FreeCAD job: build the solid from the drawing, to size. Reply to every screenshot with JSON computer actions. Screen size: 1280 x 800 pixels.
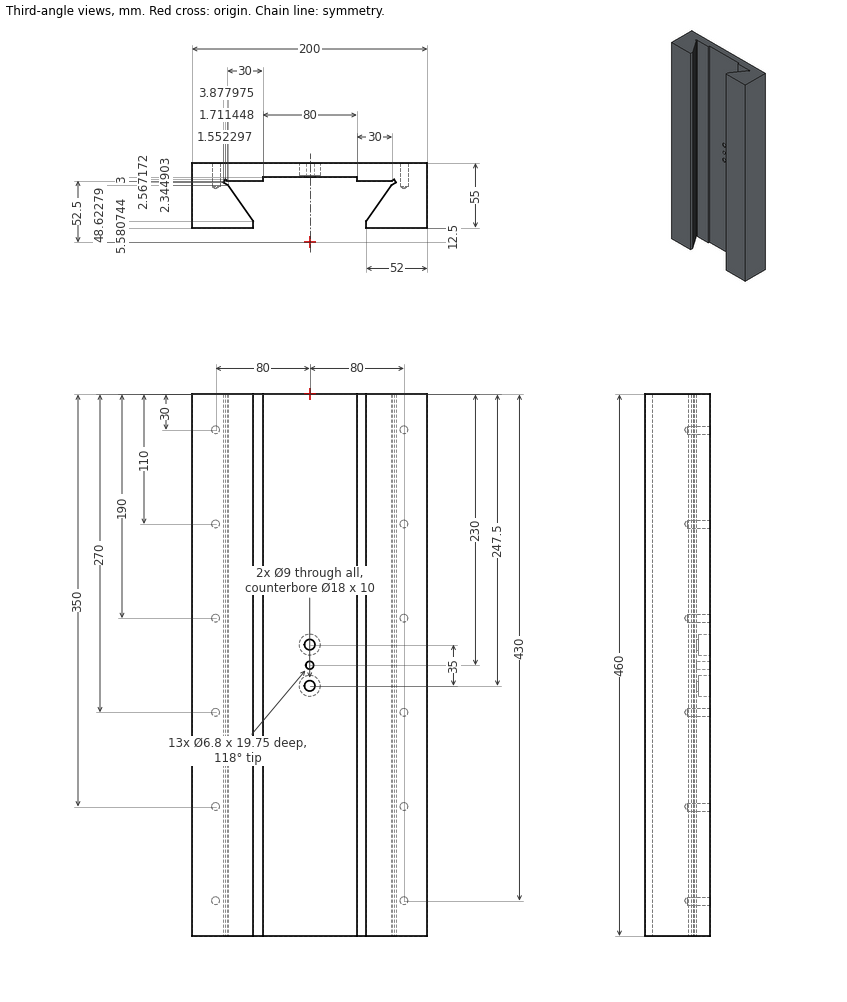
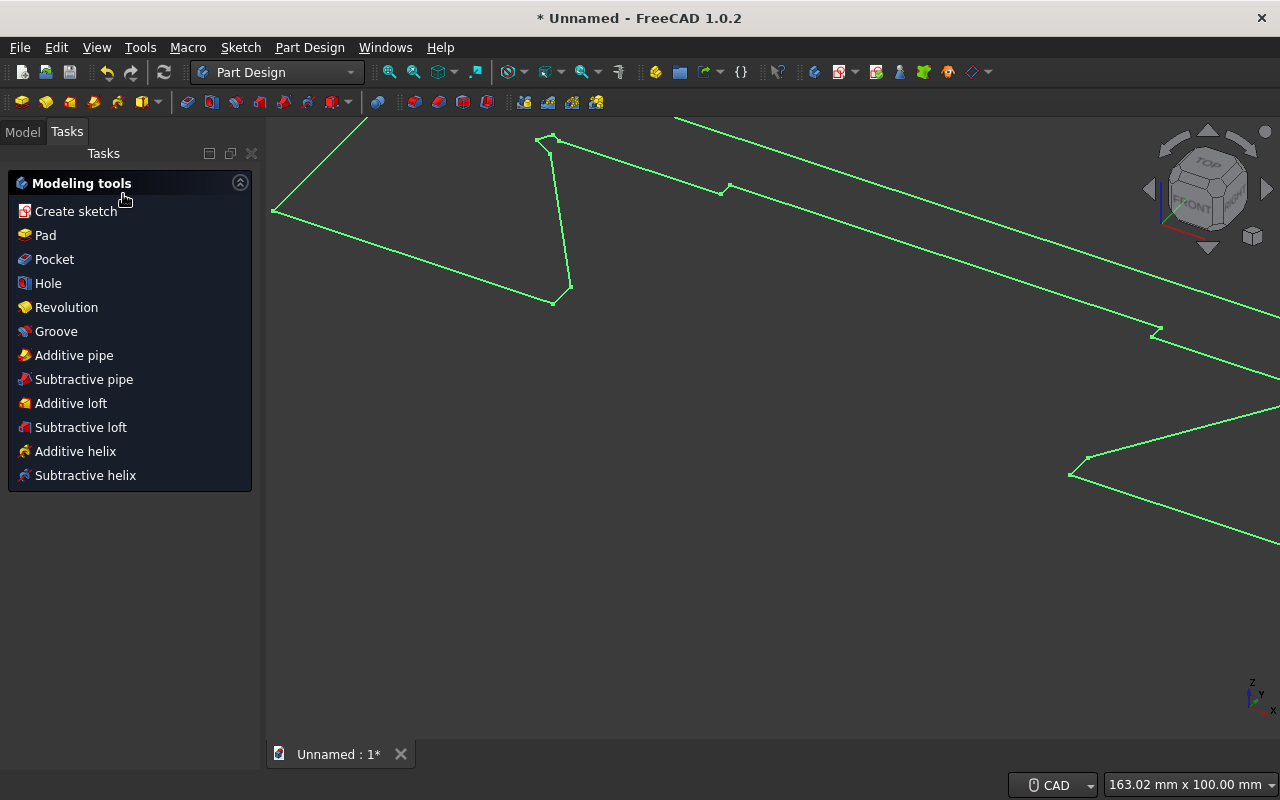
{"action": "left_click", "coordinate": [22, 102]}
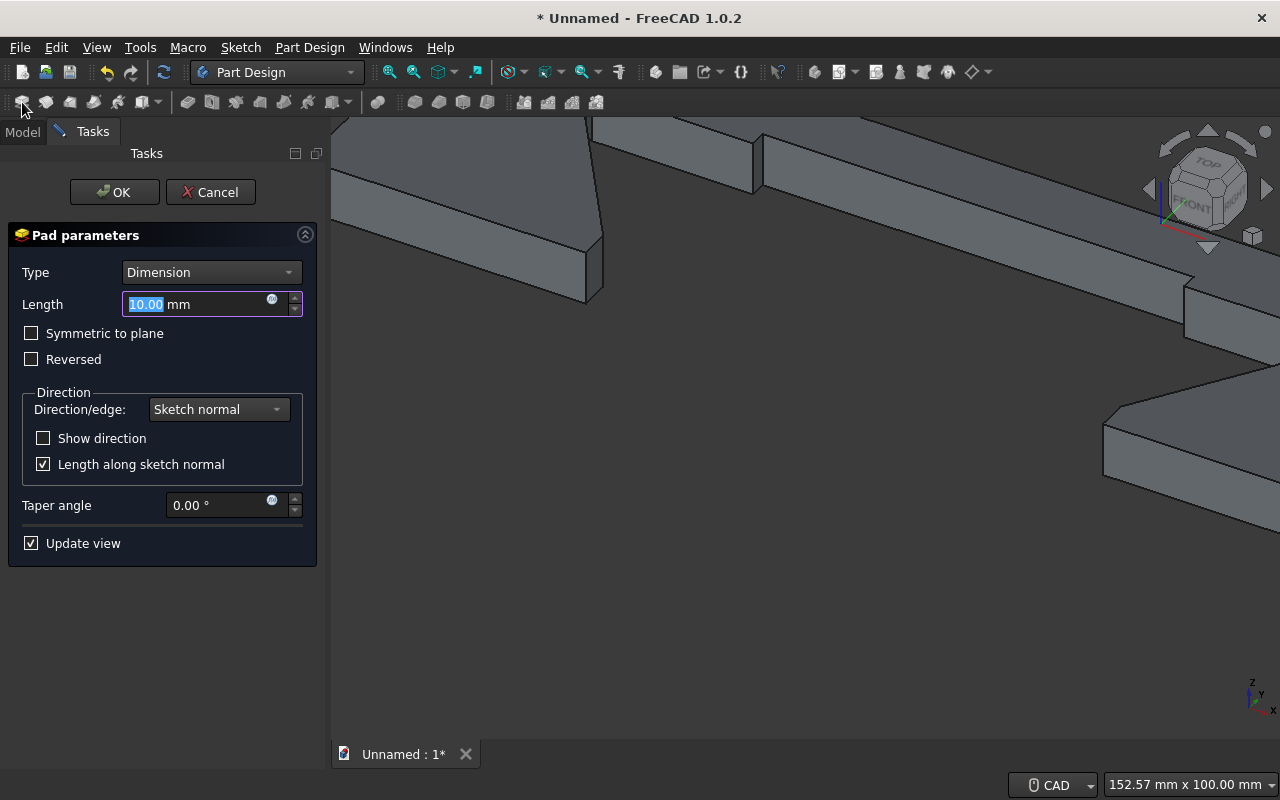
{"action": "type", "text": "460"}
{"action": "key", "text": "Tab"}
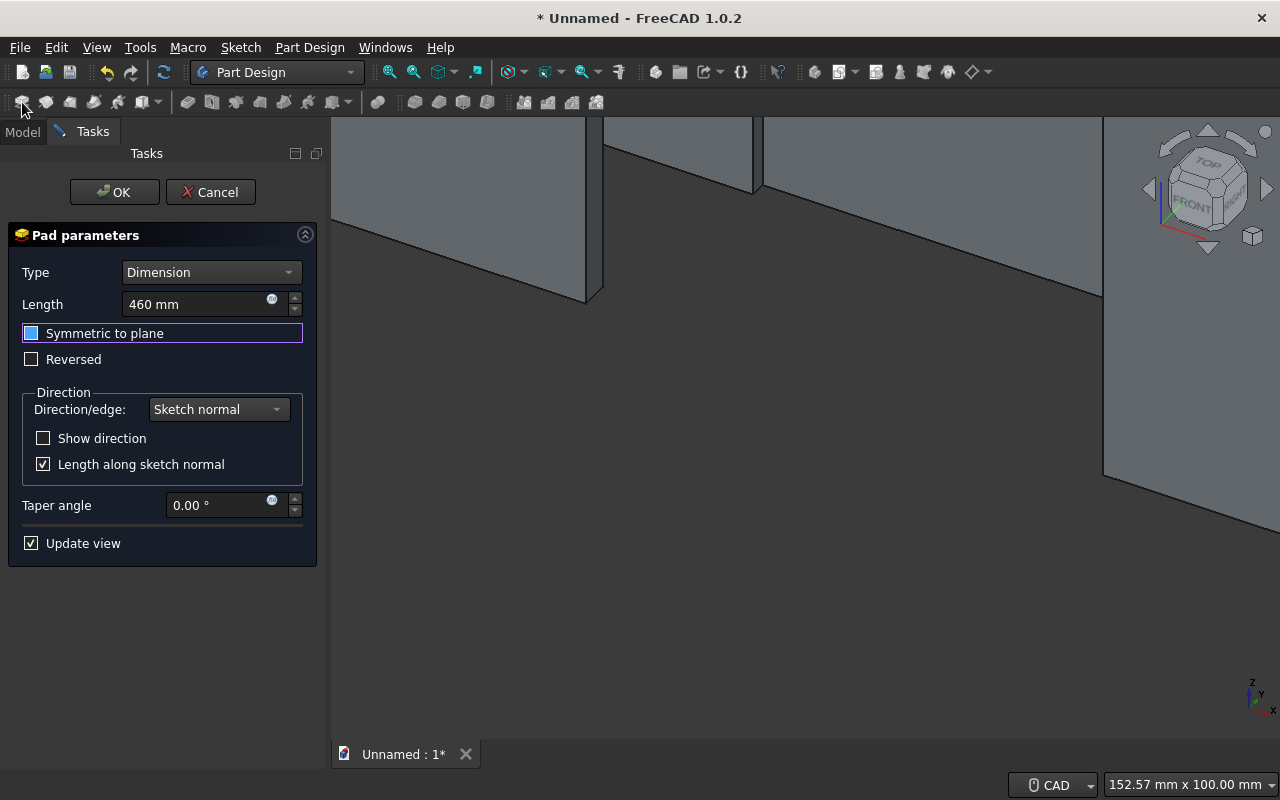
{"action": "left_click", "coordinate": [30, 359]}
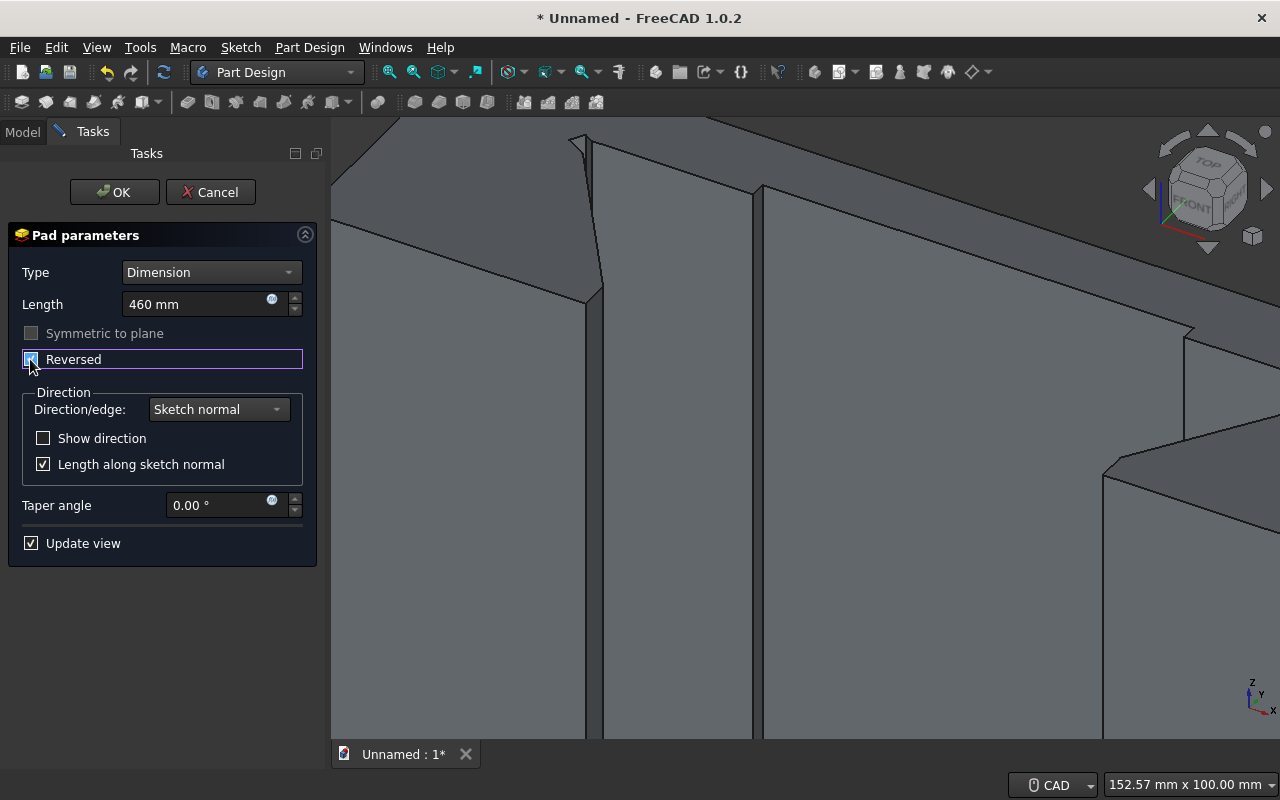
{"action": "left_click", "coordinate": [115, 192]}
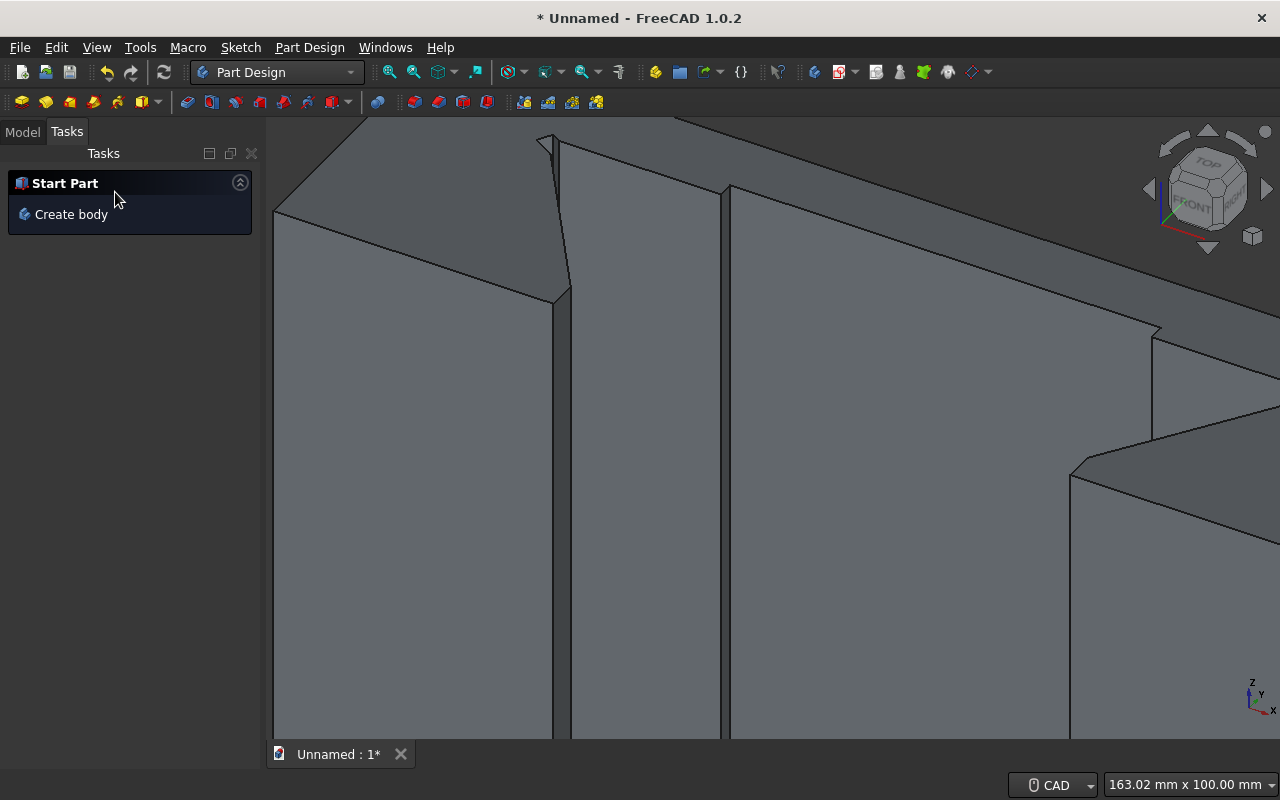
{"action": "left_click", "coordinate": [390, 72]}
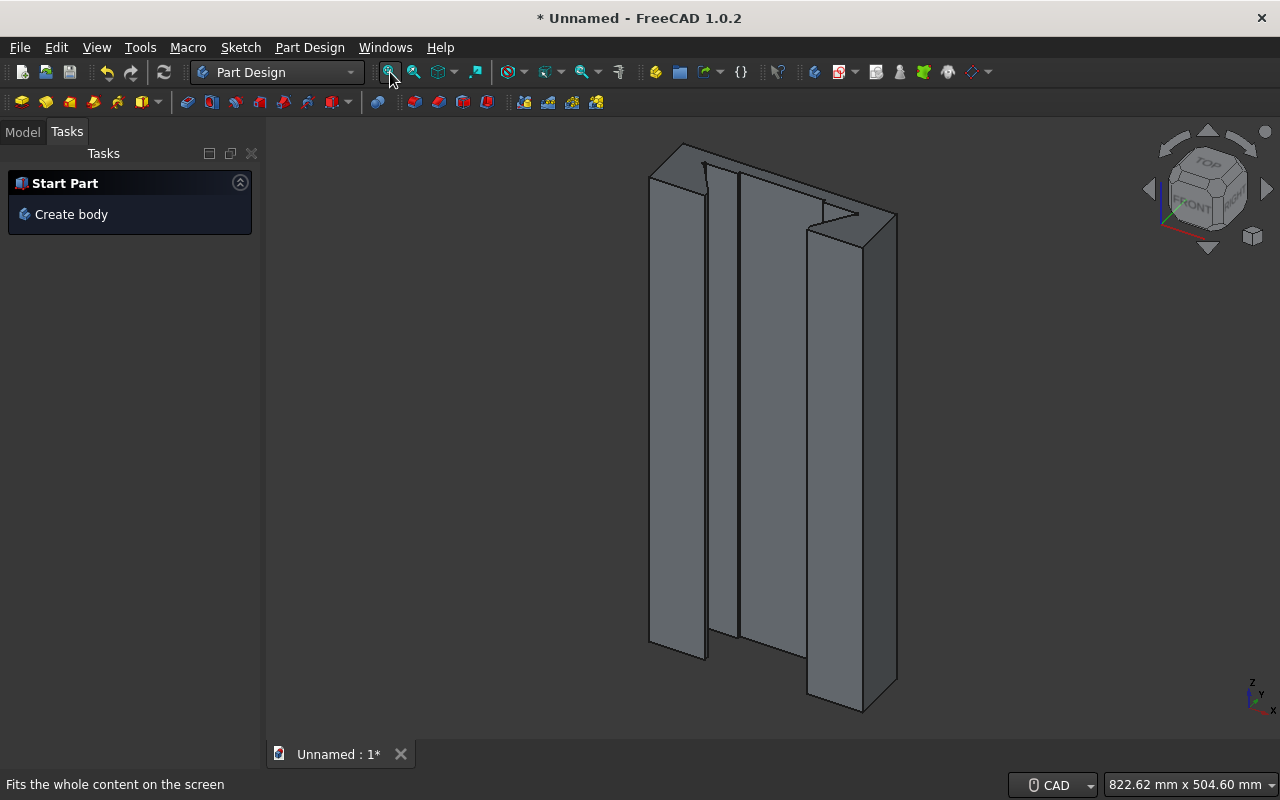
{"action": "key", "text": "4"}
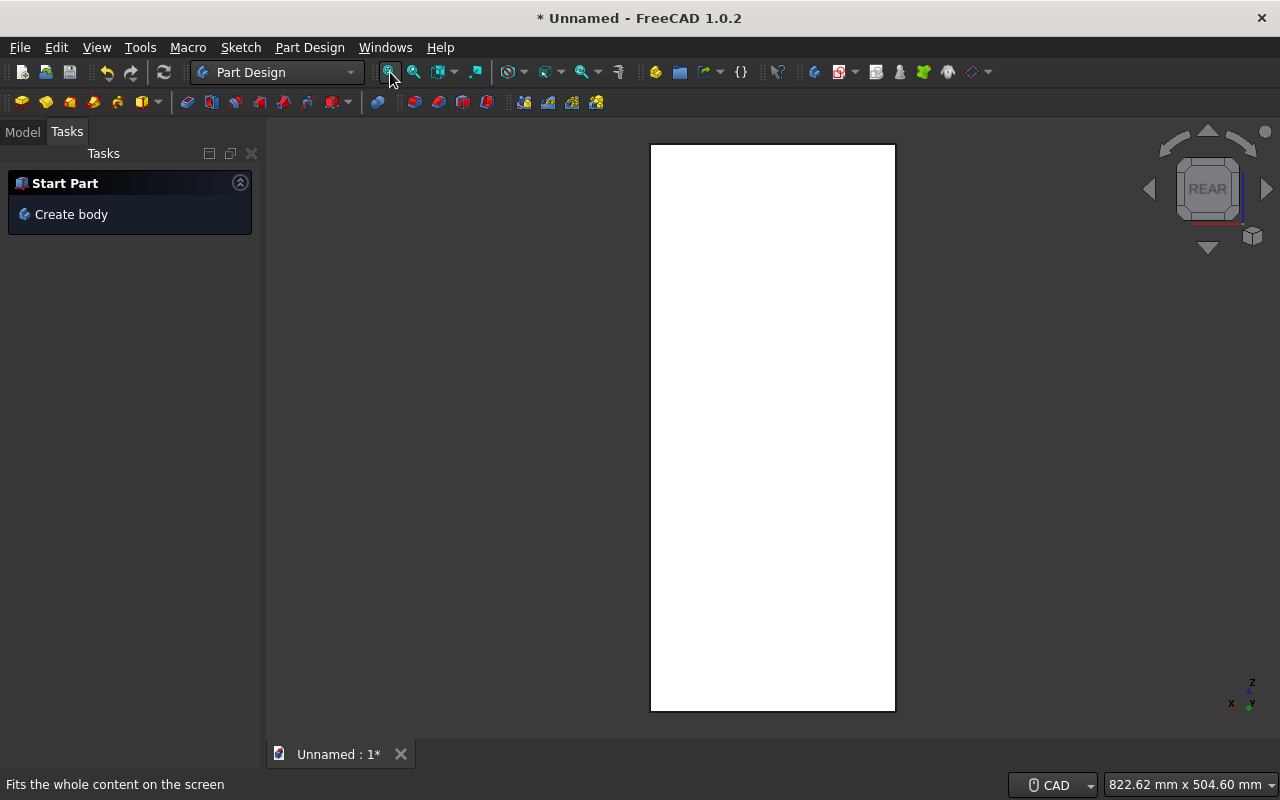
{"action": "left_click", "coordinate": [773, 346]}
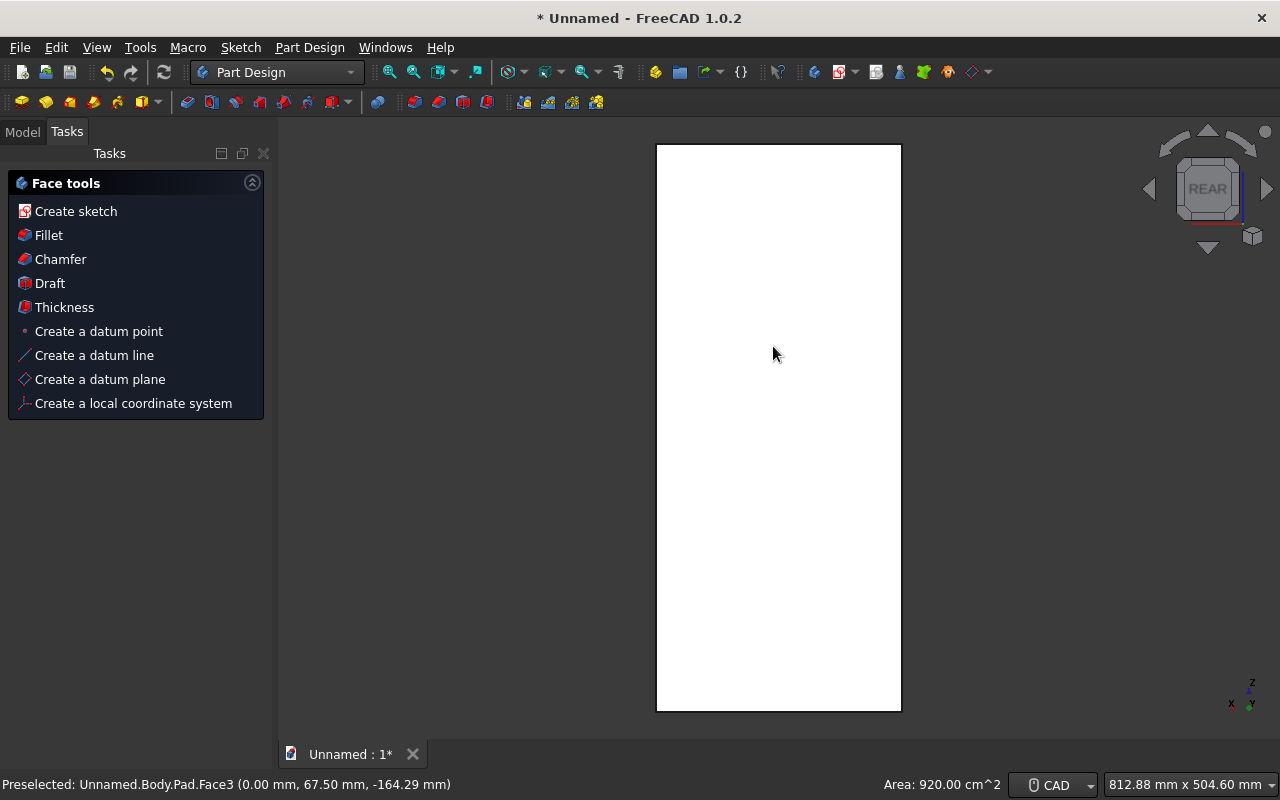
{"action": "left_click", "coordinate": [840, 72]}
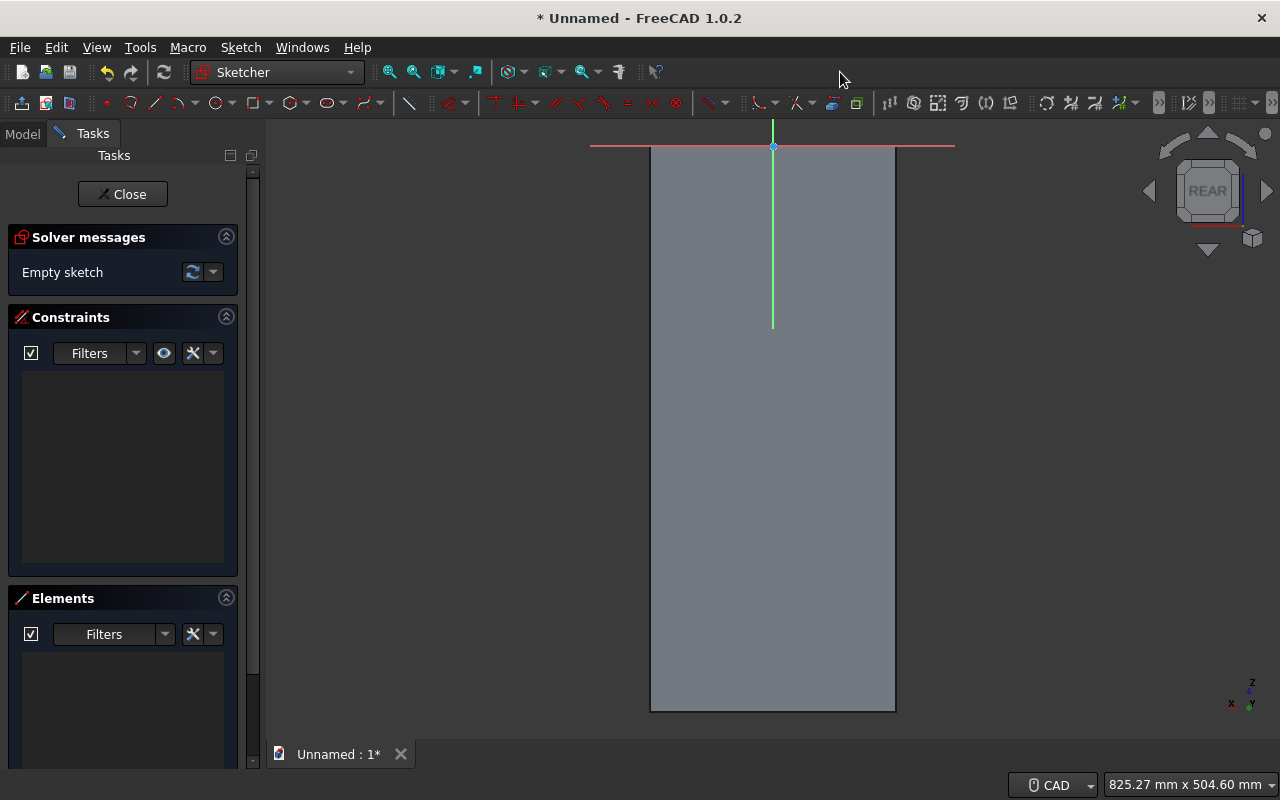
{"action": "scroll", "coordinate": [784, 429], "scroll_direction": "up", "scroll_amount": 10}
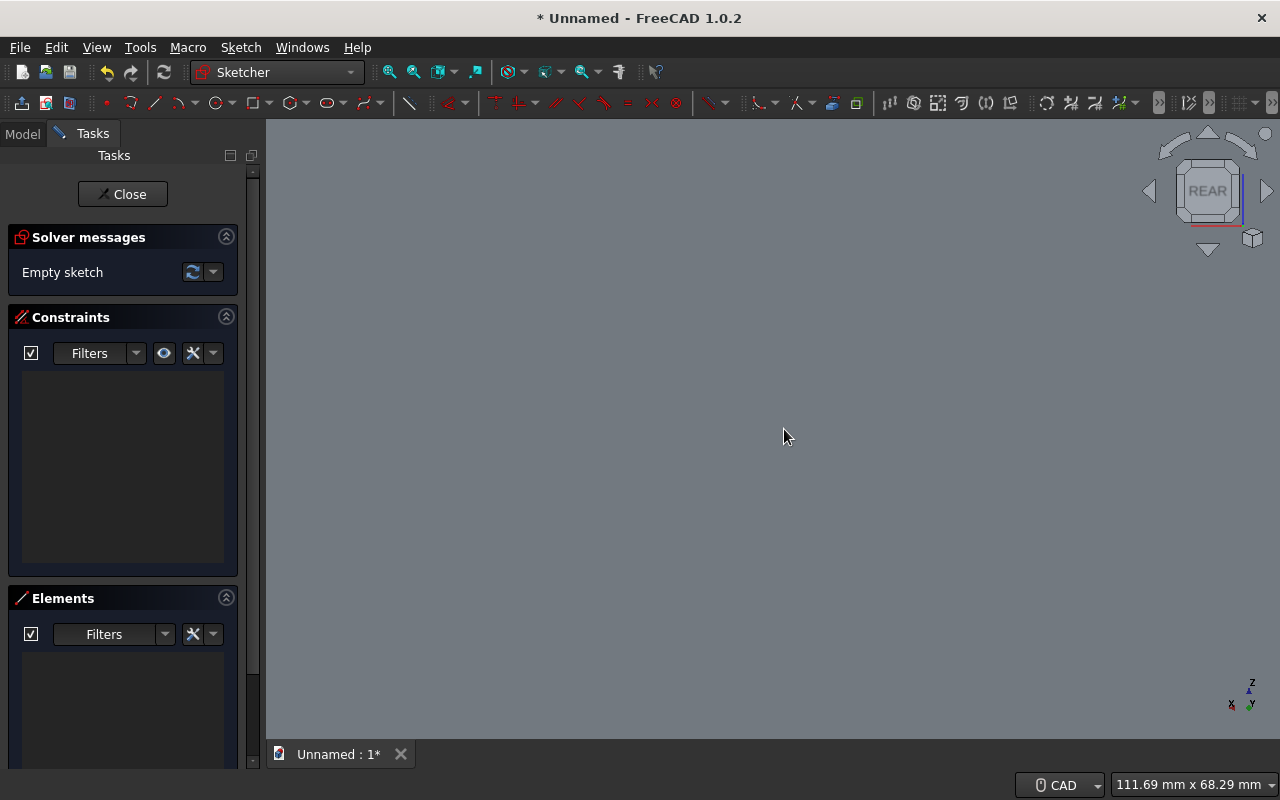
{"action": "left_click", "coordinate": [216, 104]}